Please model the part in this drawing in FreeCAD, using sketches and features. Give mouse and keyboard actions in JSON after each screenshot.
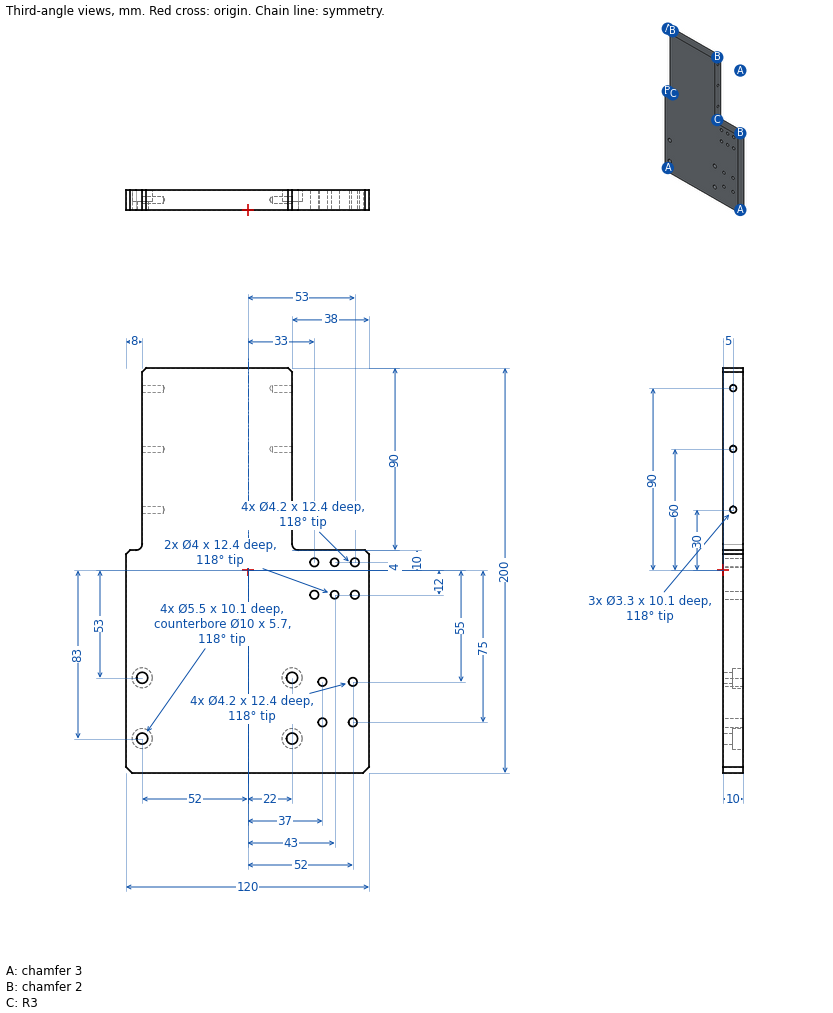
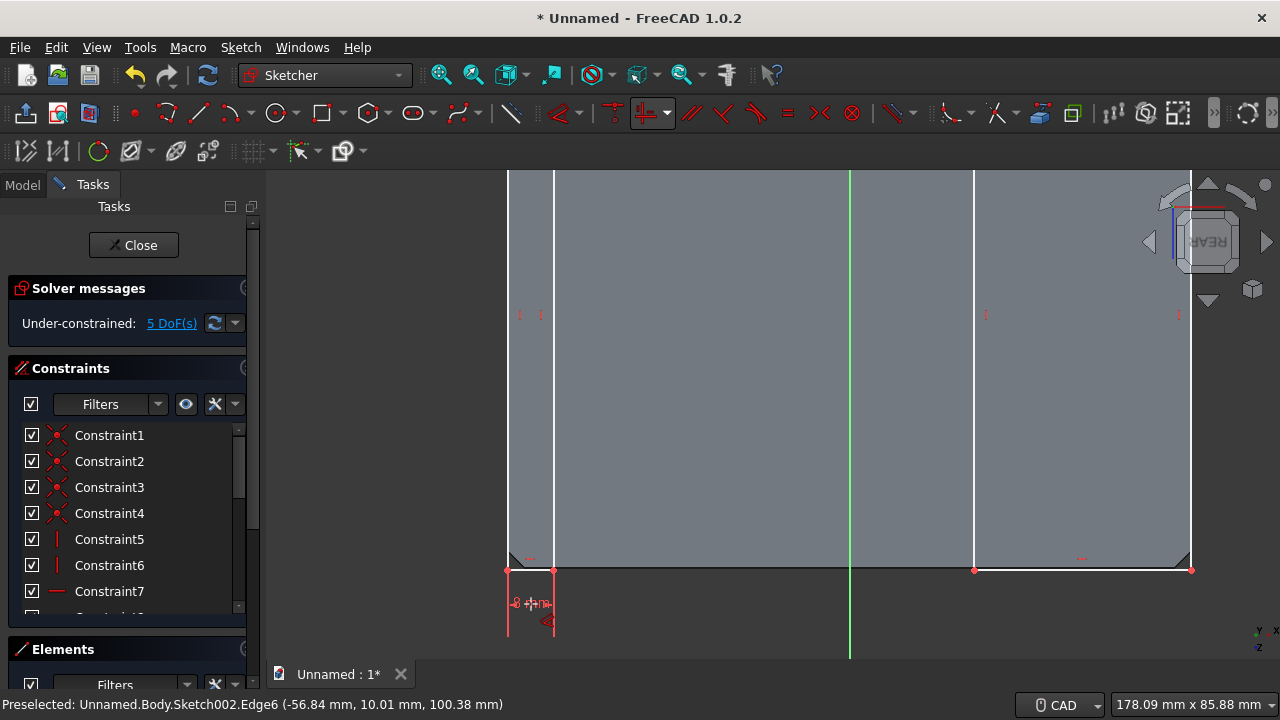
{"action": "left_click", "coordinate": [974, 212]}
{"action": "left_click", "coordinate": [1008, 384]}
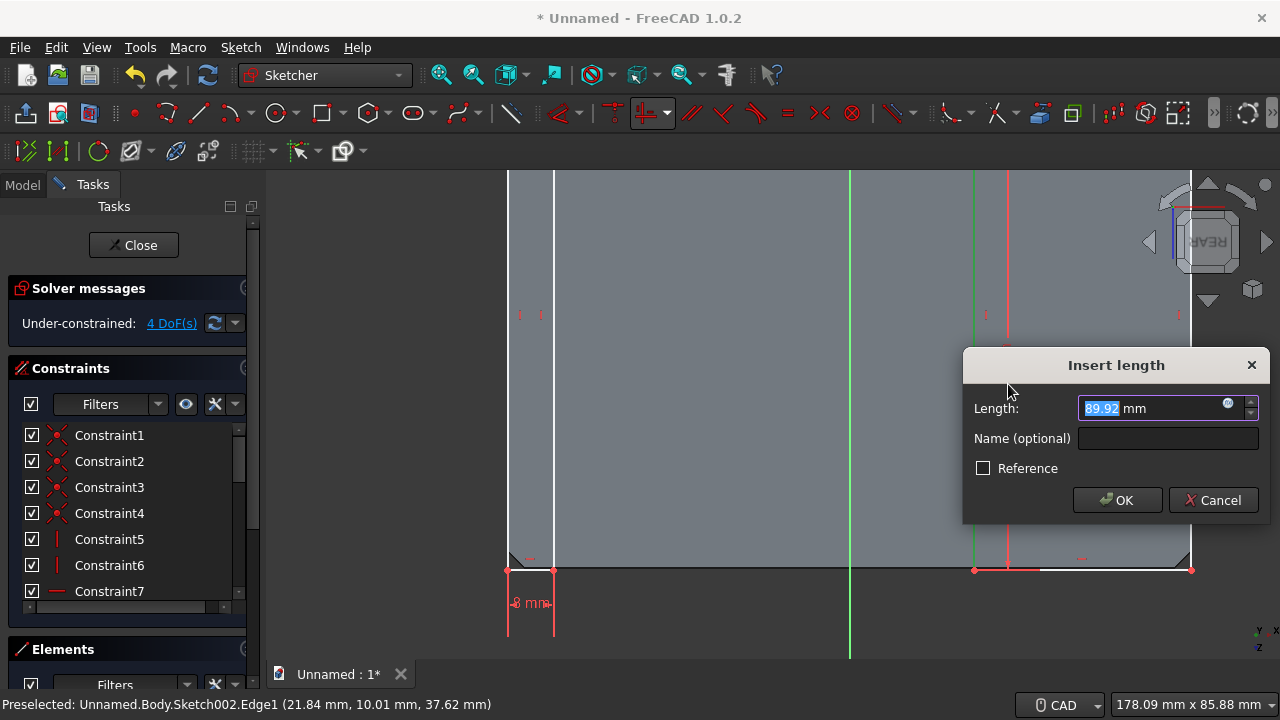
{"action": "type", "text": "90"}
{"action": "key", "text": "Return"}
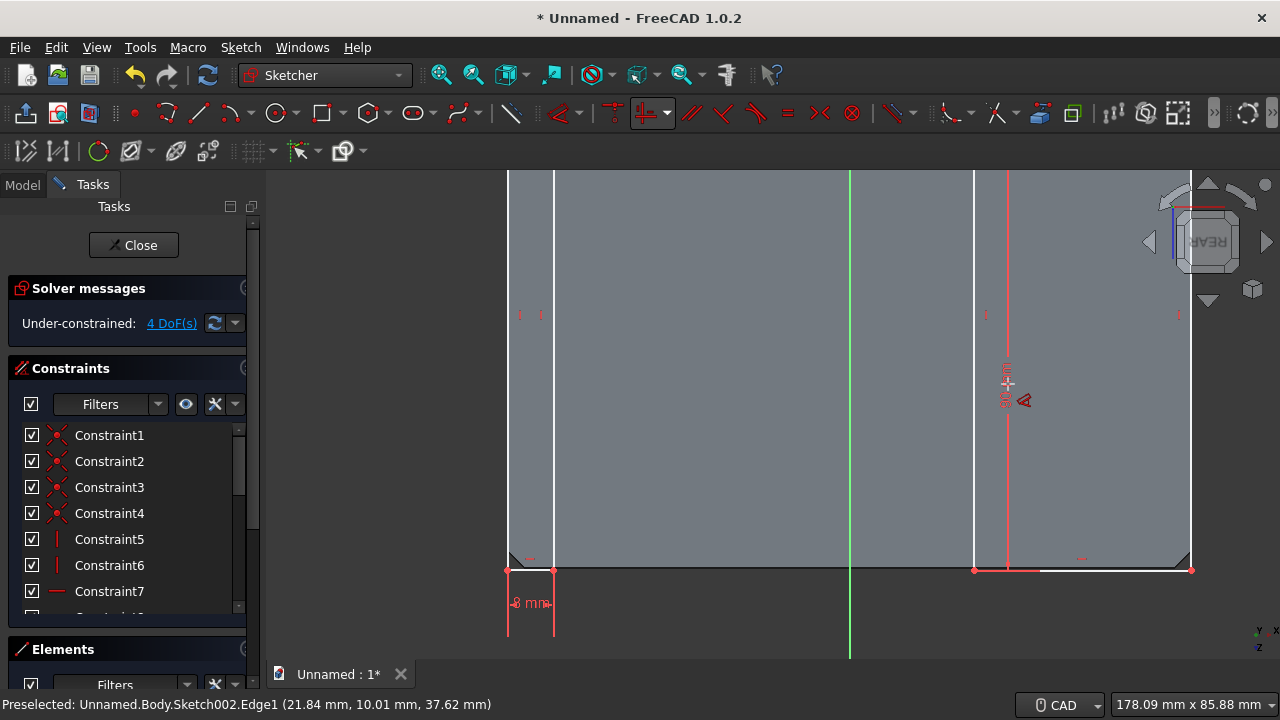
{"action": "left_click", "coordinate": [1039, 571]}
{"action": "left_click", "coordinate": [1045, 605]}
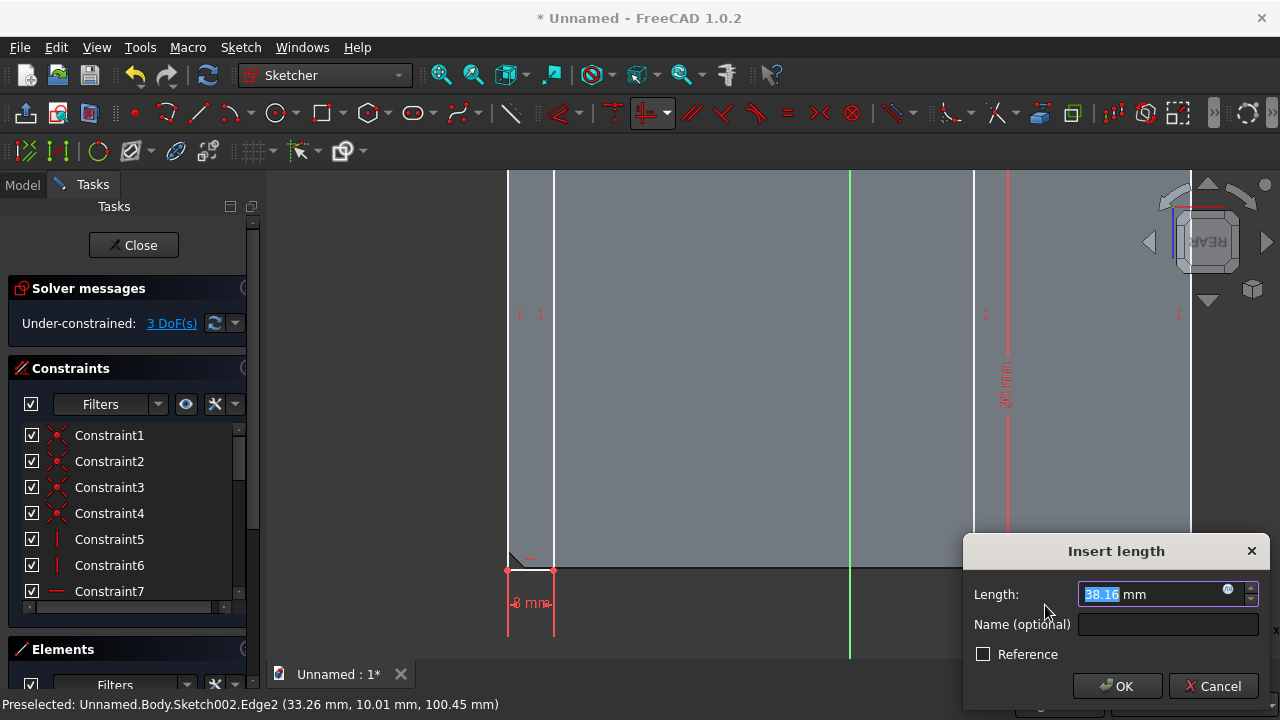
{"action": "type", "text": "38"}
{"action": "key", "text": "Return"}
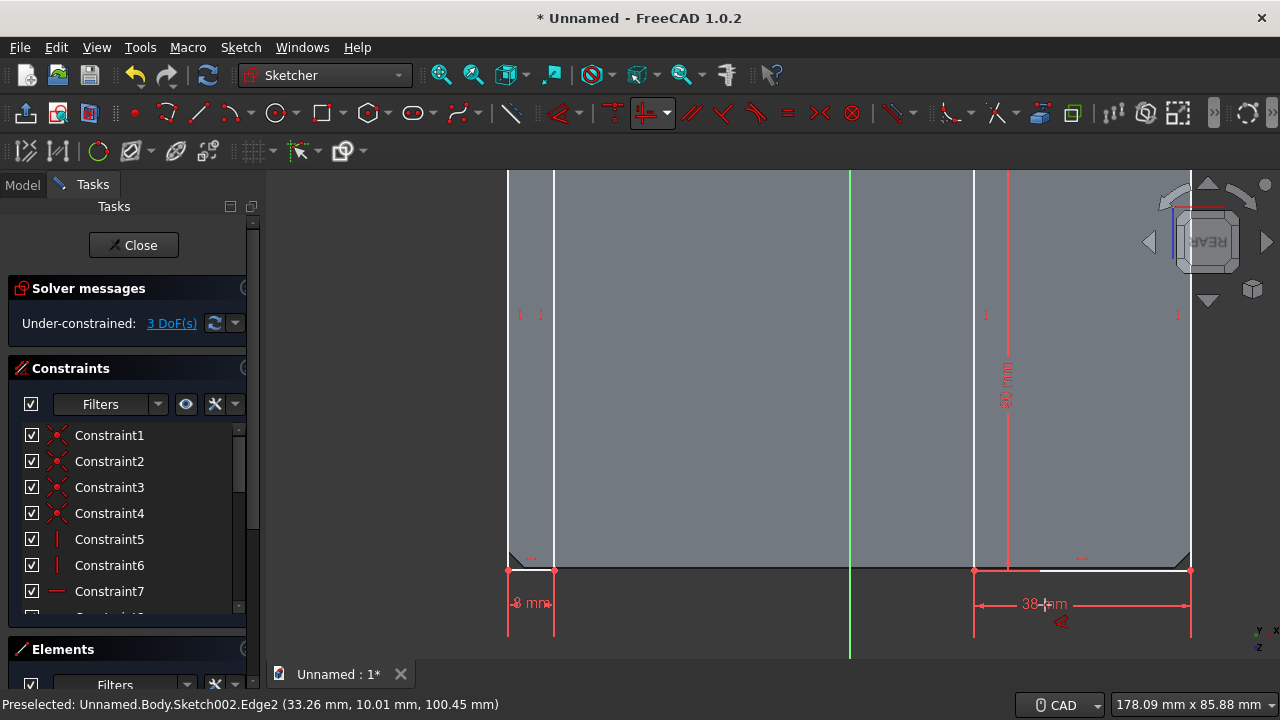
{"action": "left_click", "coordinate": [509, 212]}
{"action": "left_click", "coordinate": [475, 384]}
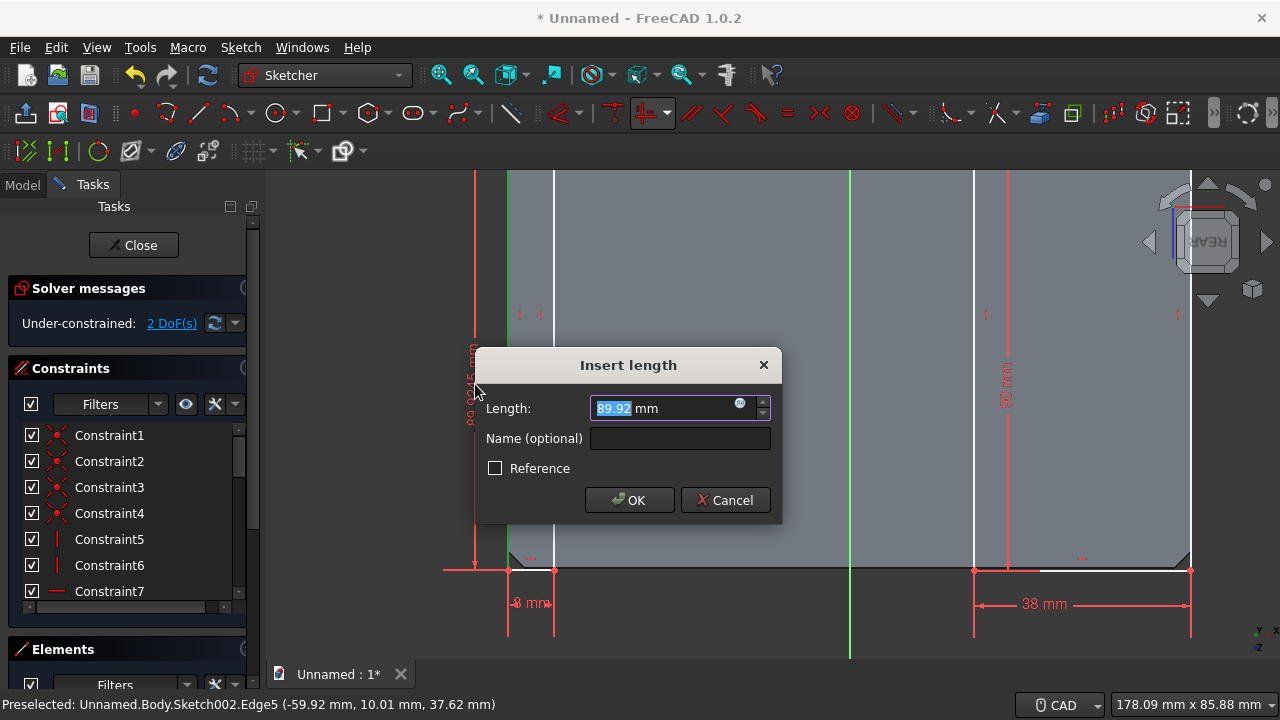
{"action": "type", "text": "90"}
{"action": "key", "text": "Return"}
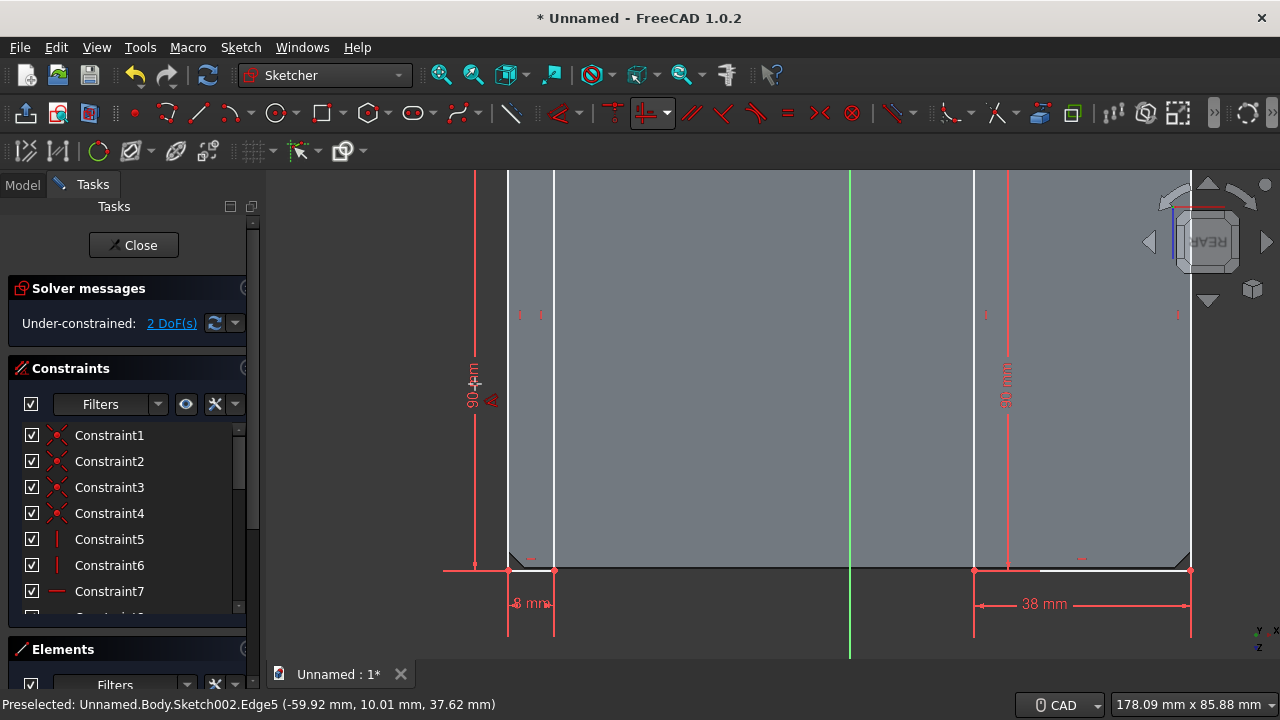
{"action": "scroll", "coordinate": [528, 574], "scroll_direction": "down", "scroll_amount": 3}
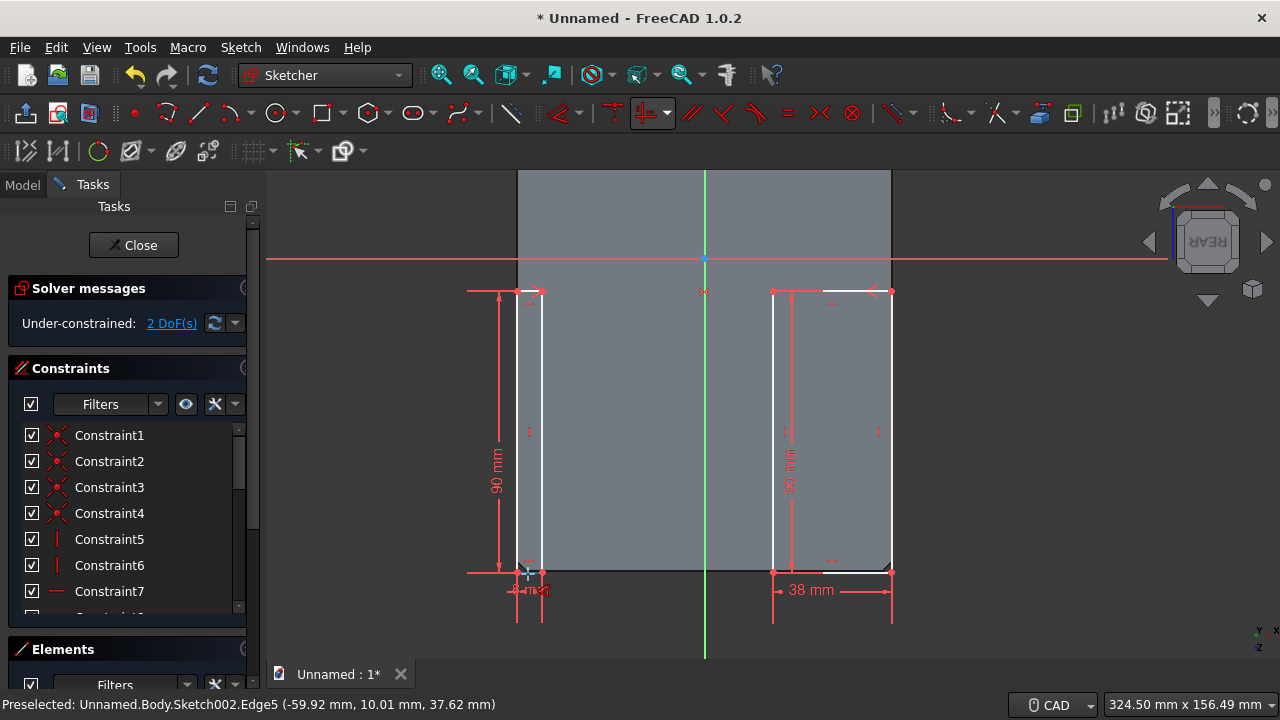
{"action": "left_click", "coordinate": [773, 291]}
{"action": "left_click", "coordinate": [739, 225]}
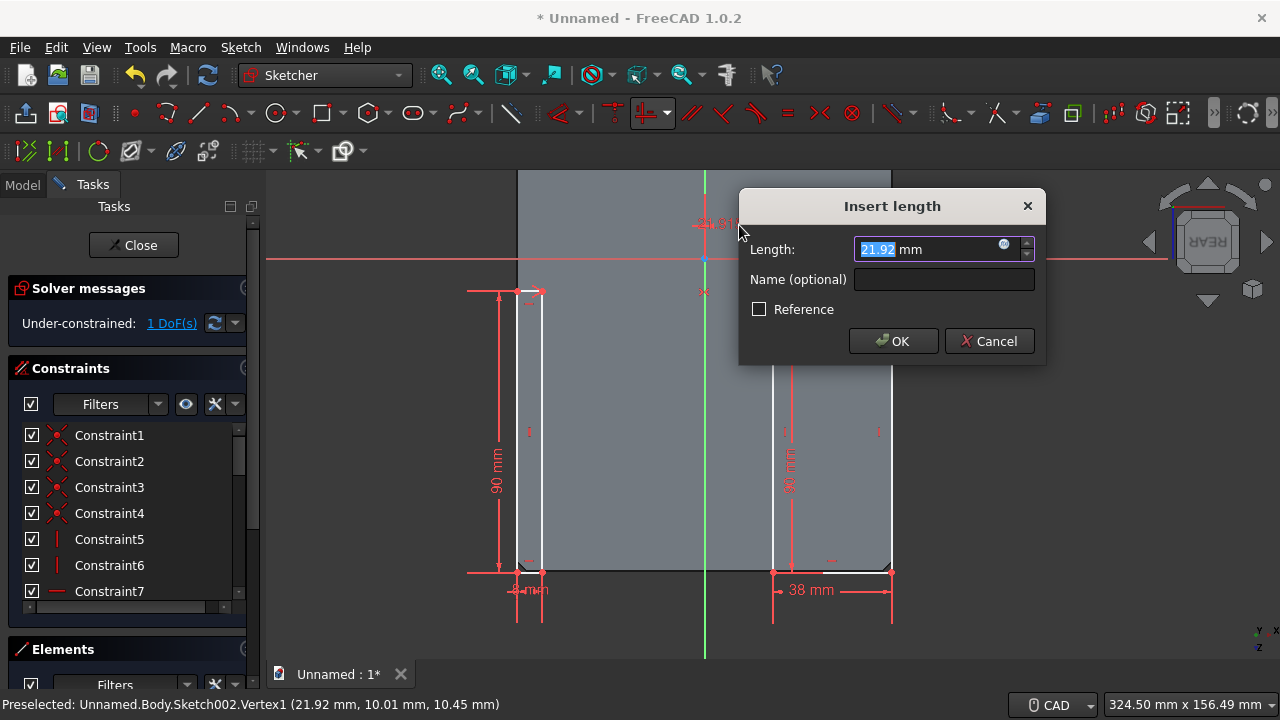
{"action": "type", "text": "22"}
{"action": "key", "text": "Return"}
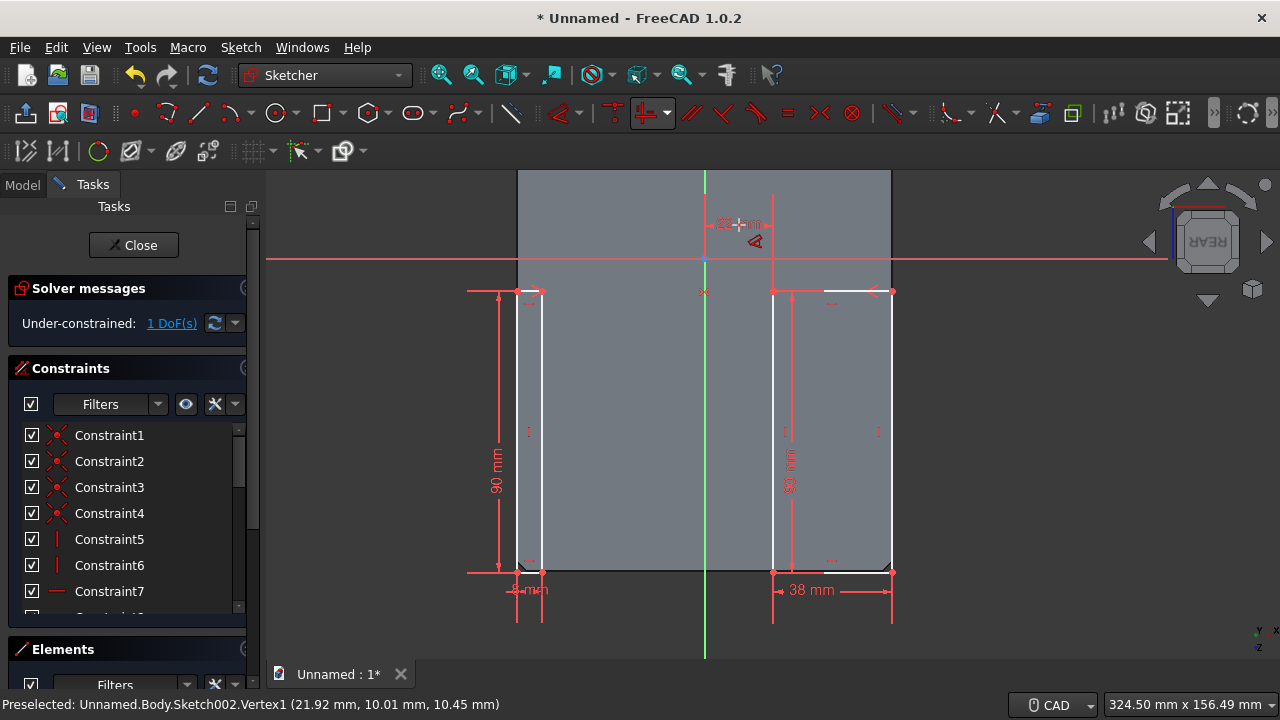
{"action": "scroll", "coordinate": [773, 291], "scroll_direction": "up", "scroll_amount": 2}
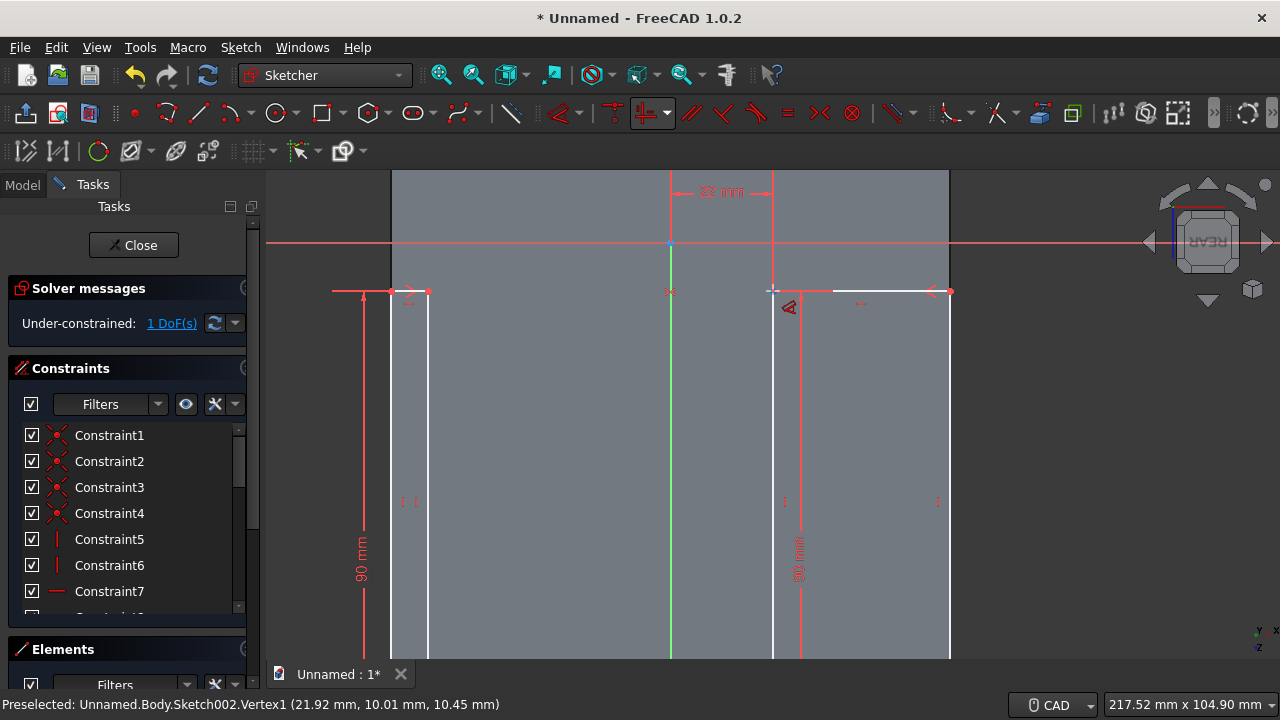
{"action": "left_click", "coordinate": [773, 291]}
{"action": "left_click", "coordinate": [807, 267]}